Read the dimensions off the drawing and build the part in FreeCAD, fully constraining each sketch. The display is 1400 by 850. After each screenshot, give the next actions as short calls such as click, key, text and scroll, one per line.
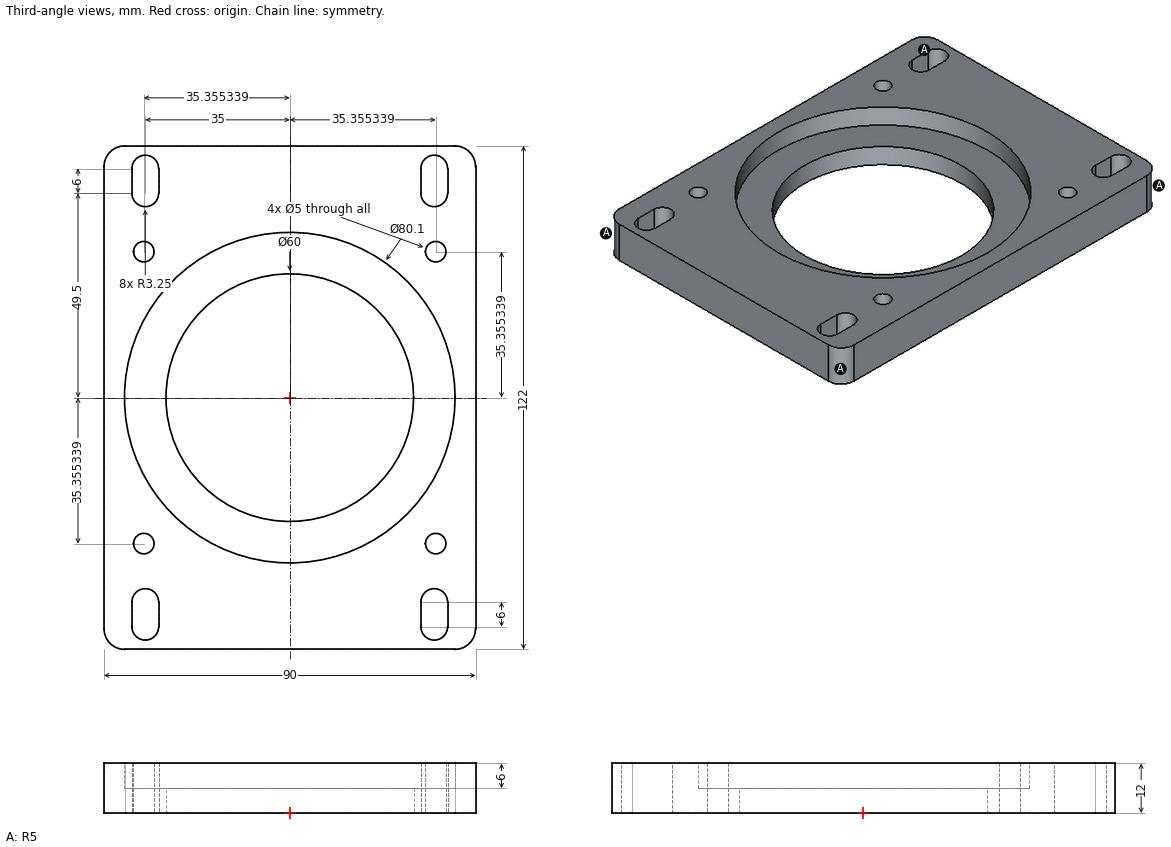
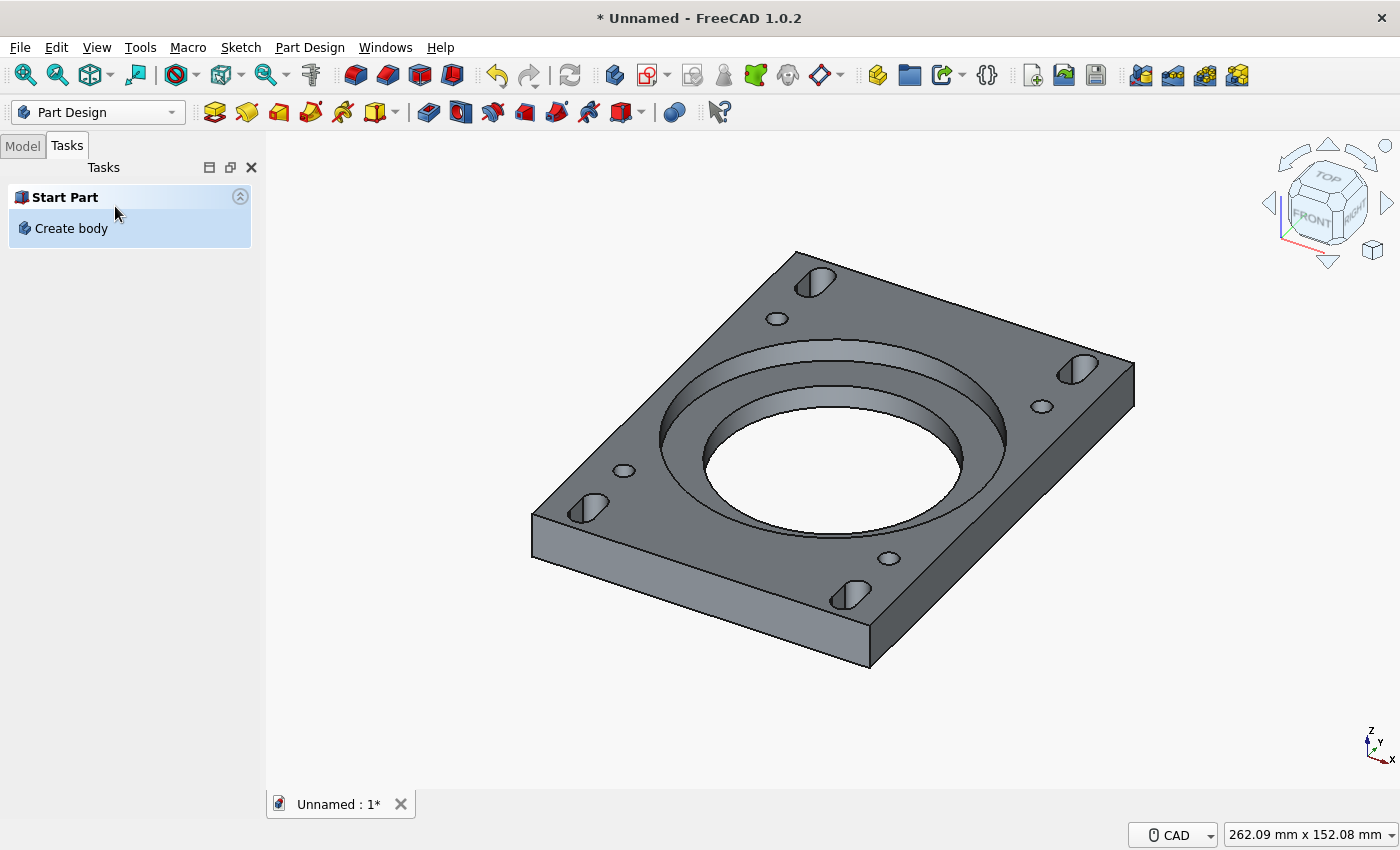
click(870, 646)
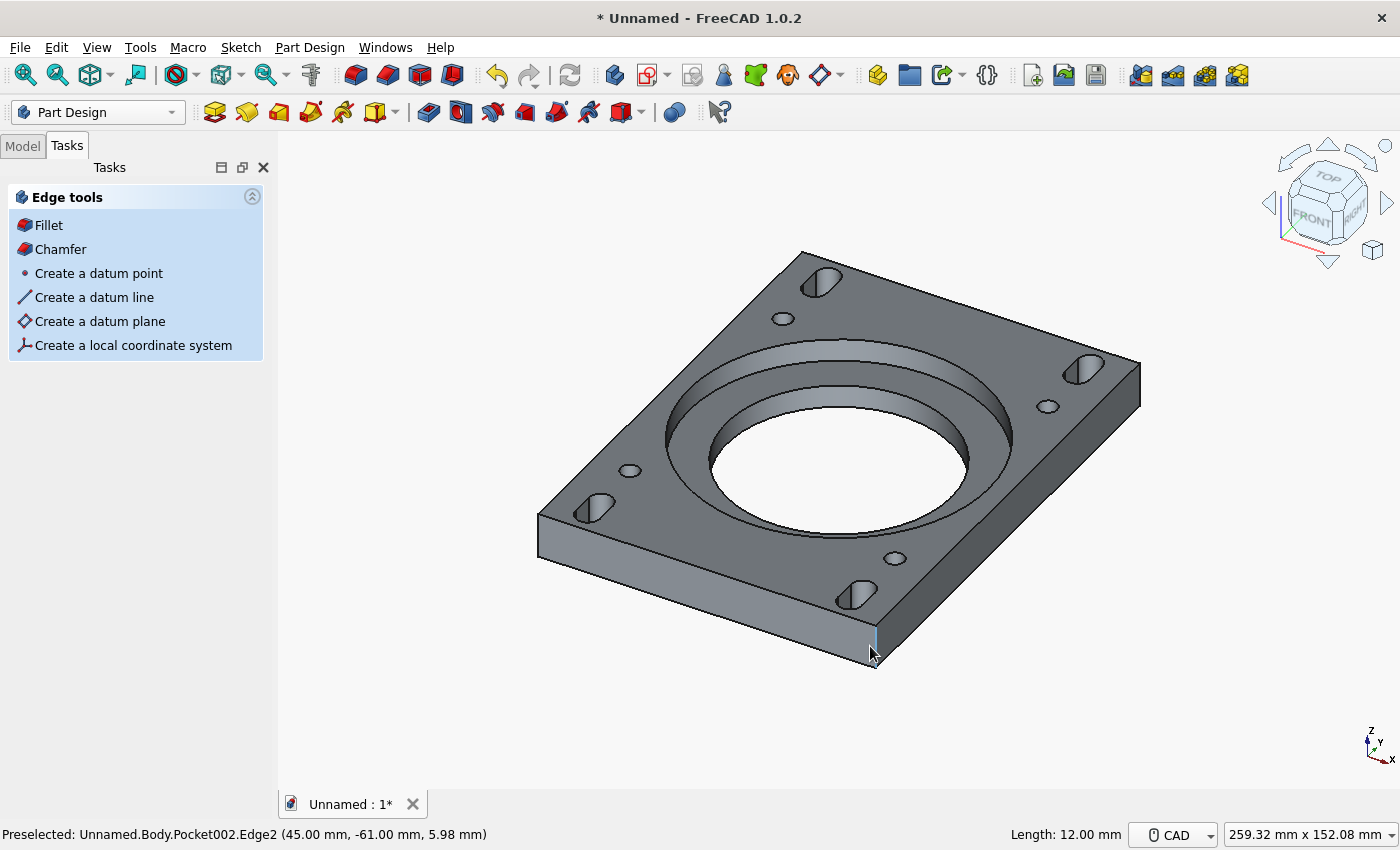
key(0)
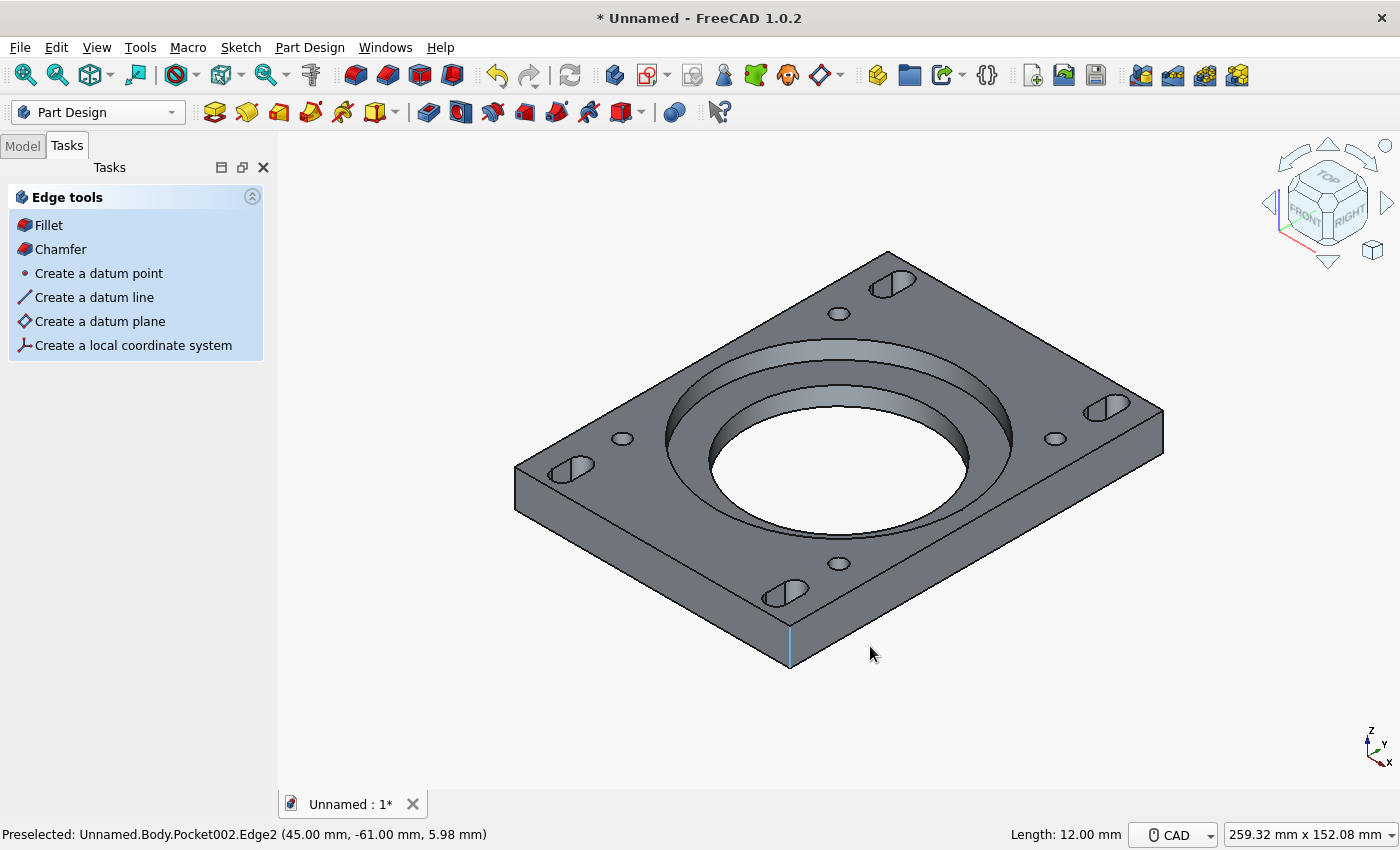
key(2)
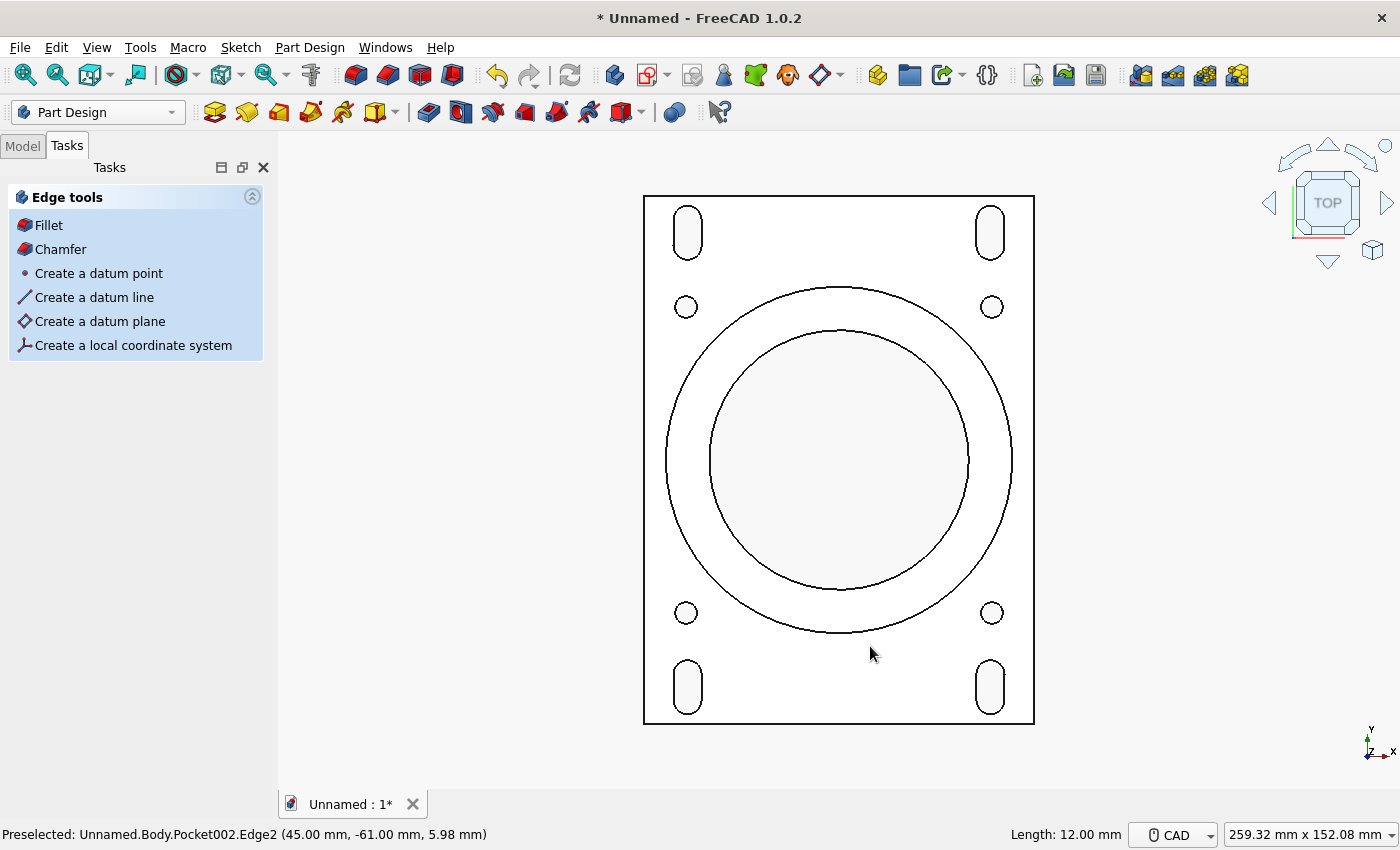
key(1)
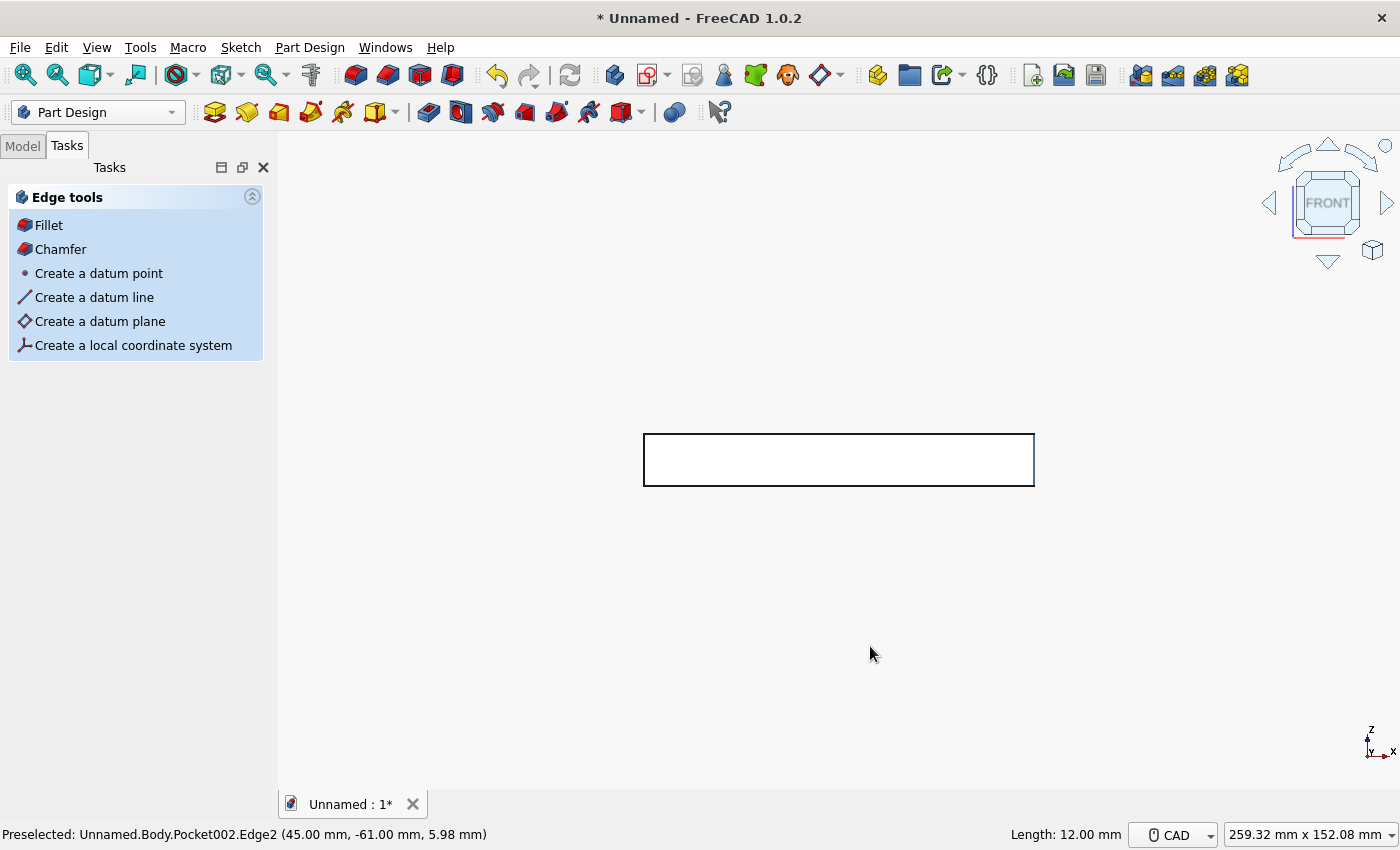
click(26, 76)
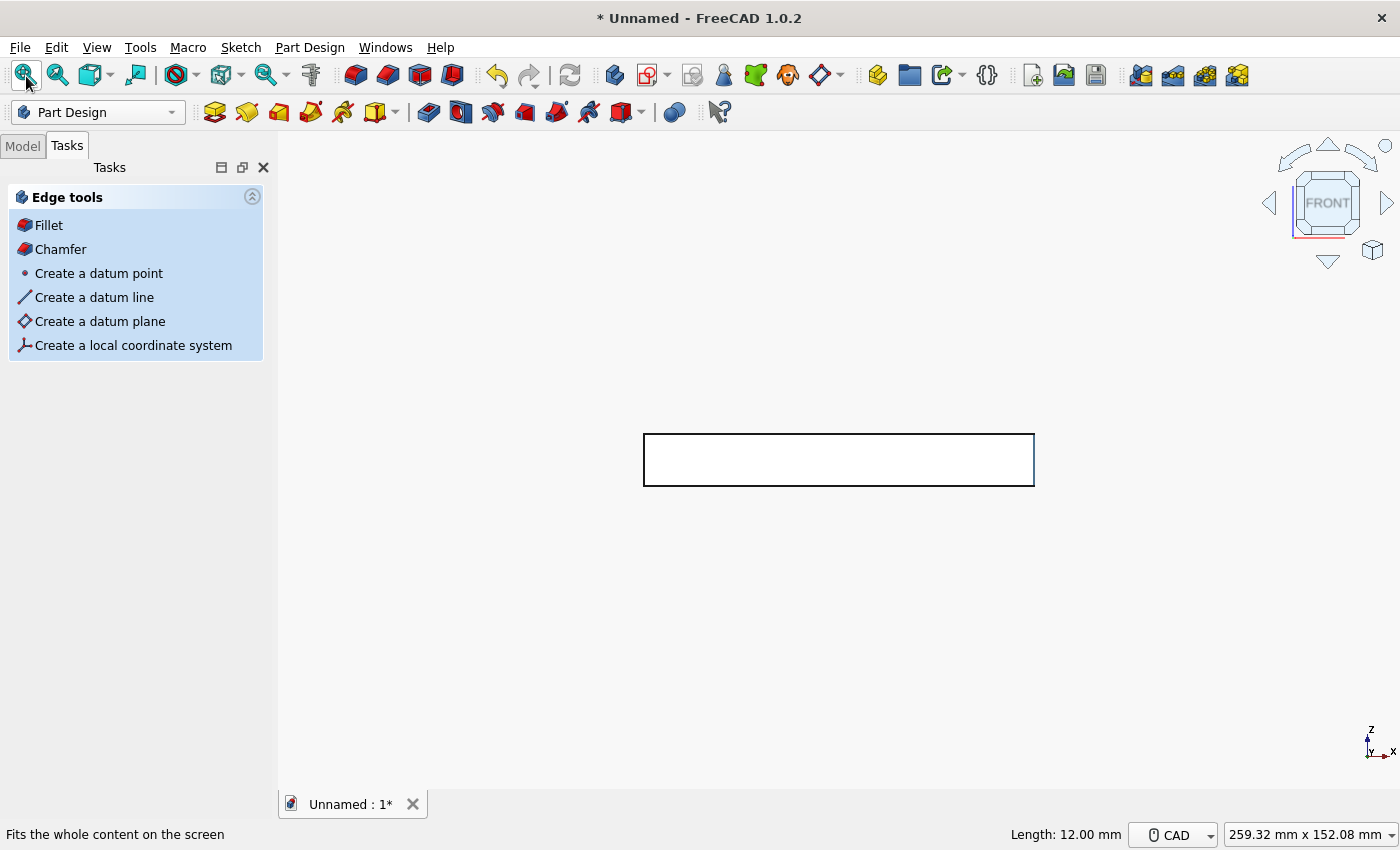
click(644, 459, ctrl)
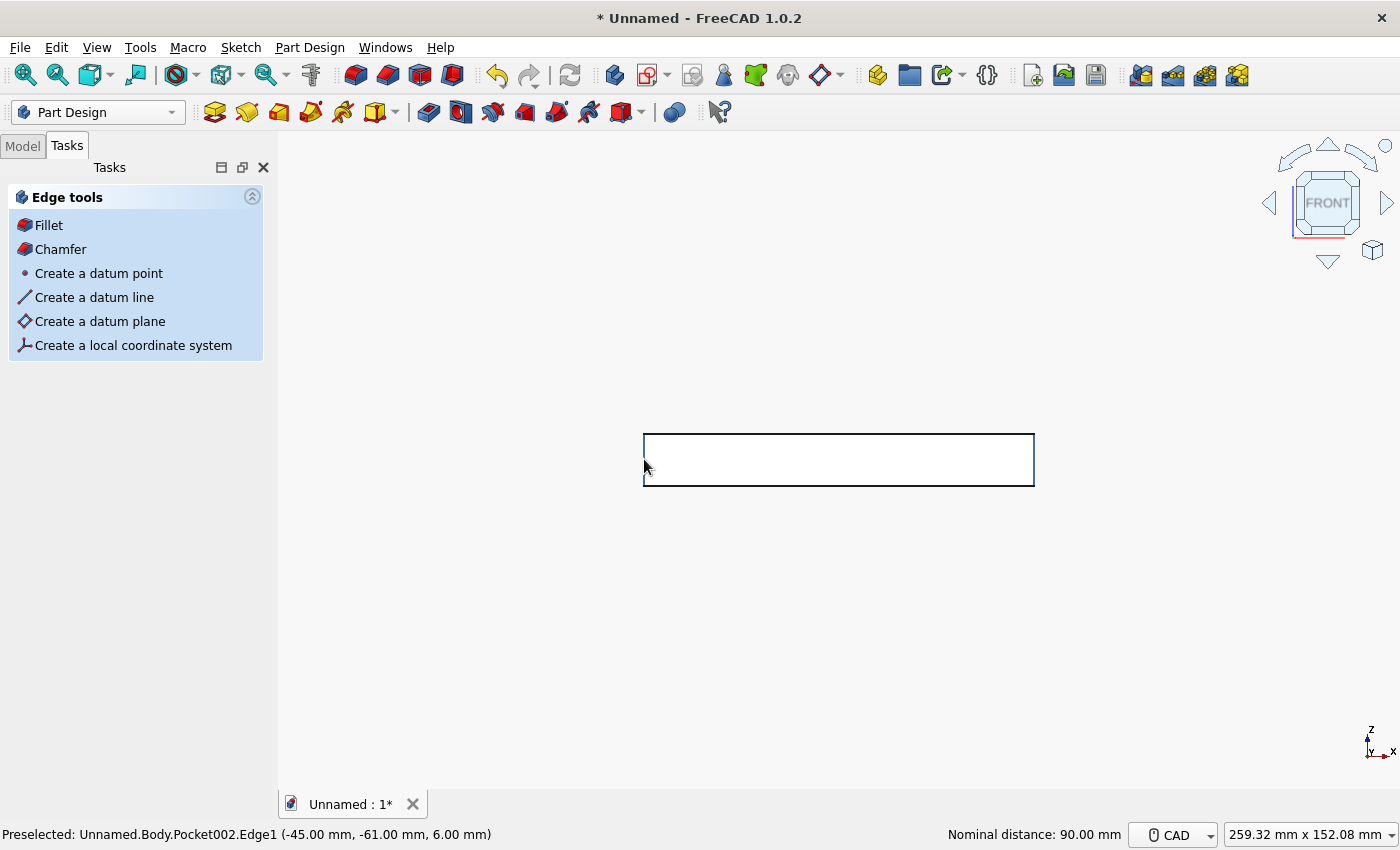
key(3)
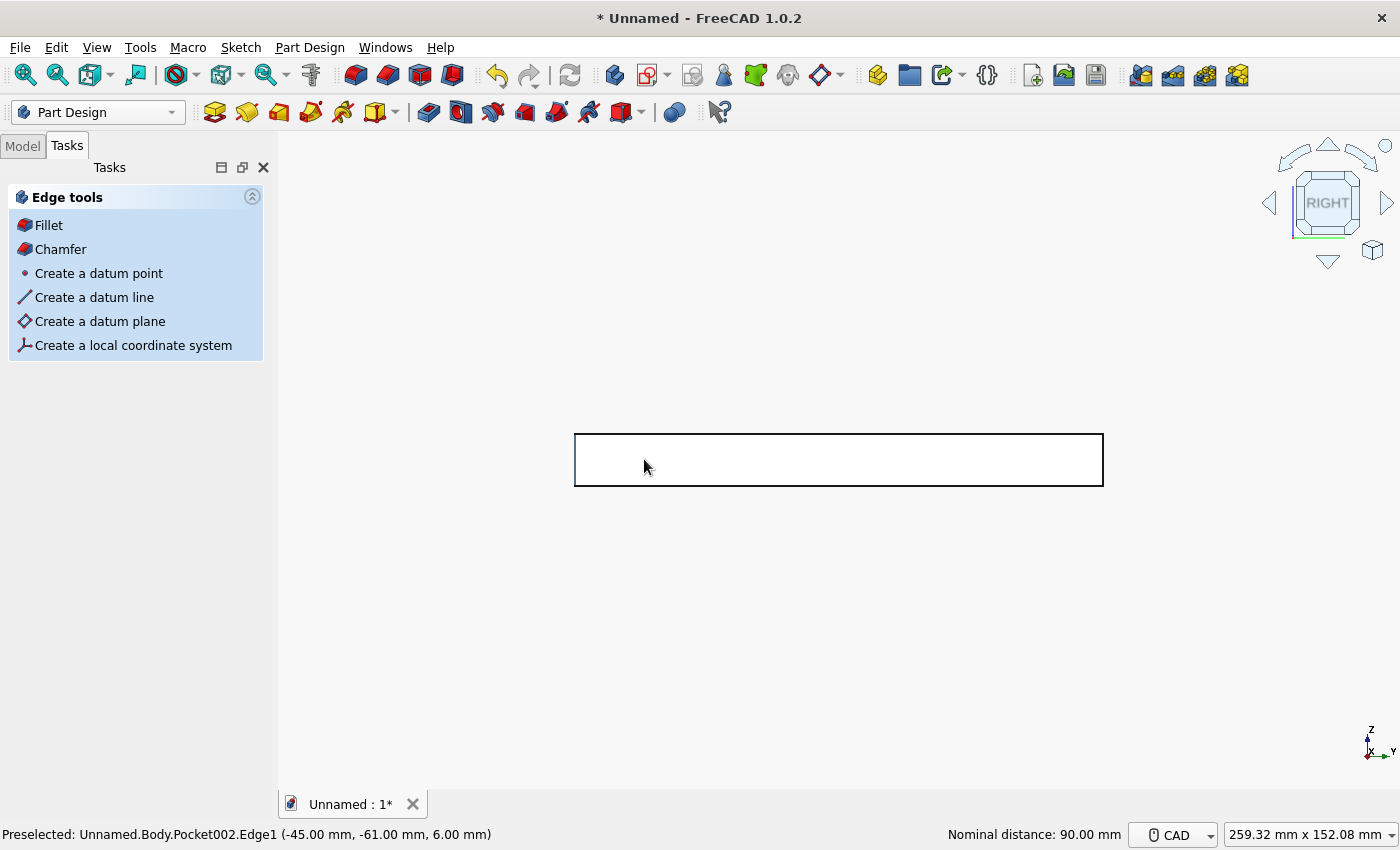
click(1103, 459, ctrl)